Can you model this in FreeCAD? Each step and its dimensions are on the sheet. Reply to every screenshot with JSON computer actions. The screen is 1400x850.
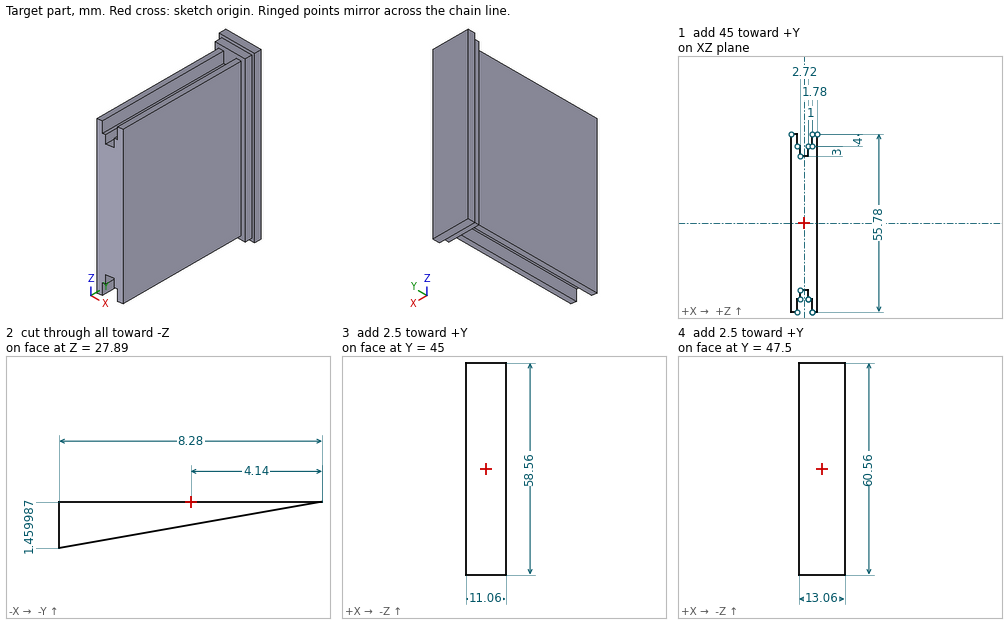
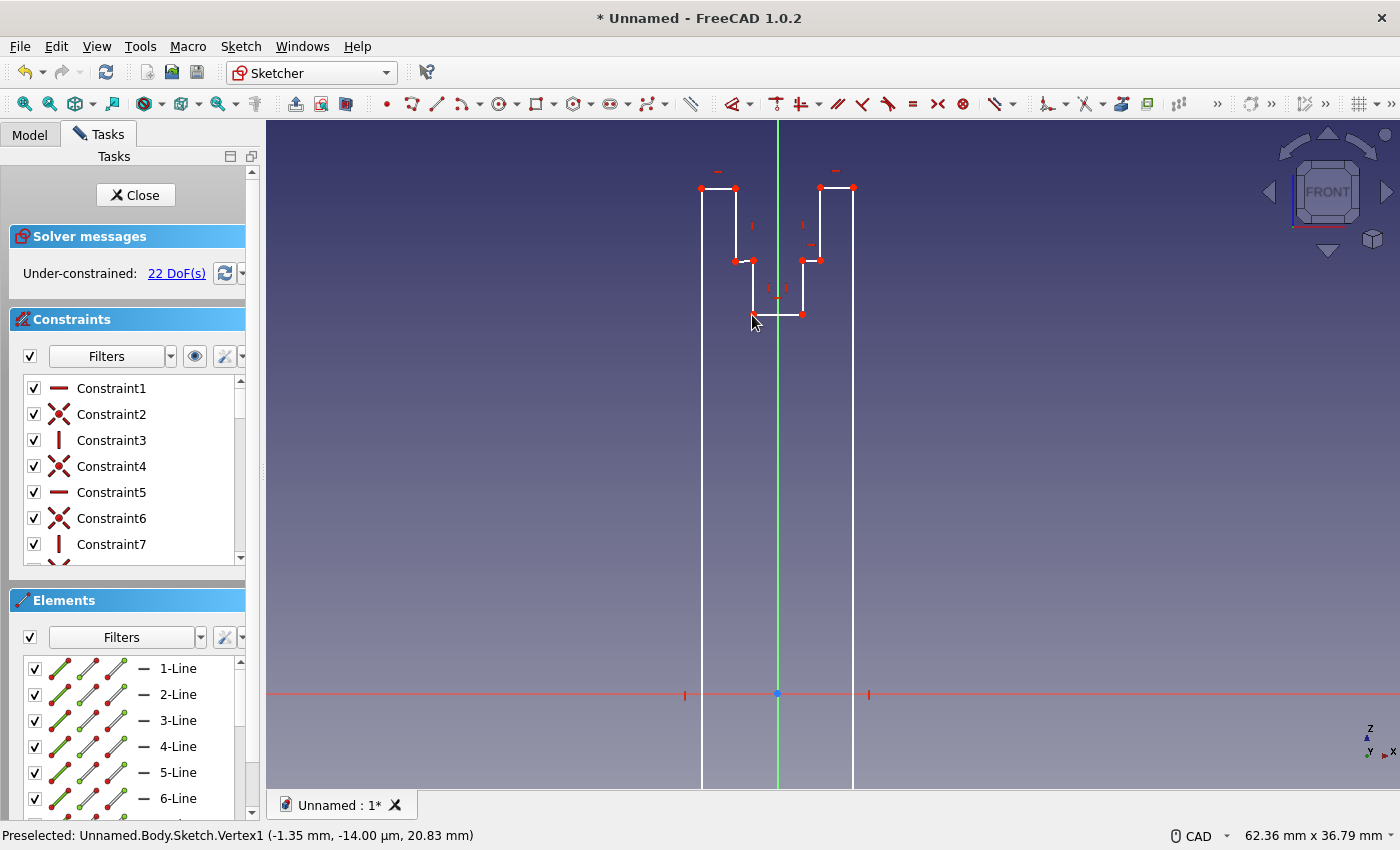
{"action": "scroll", "coordinate": [754, 259], "scroll_direction": "down", "scroll_amount": 4}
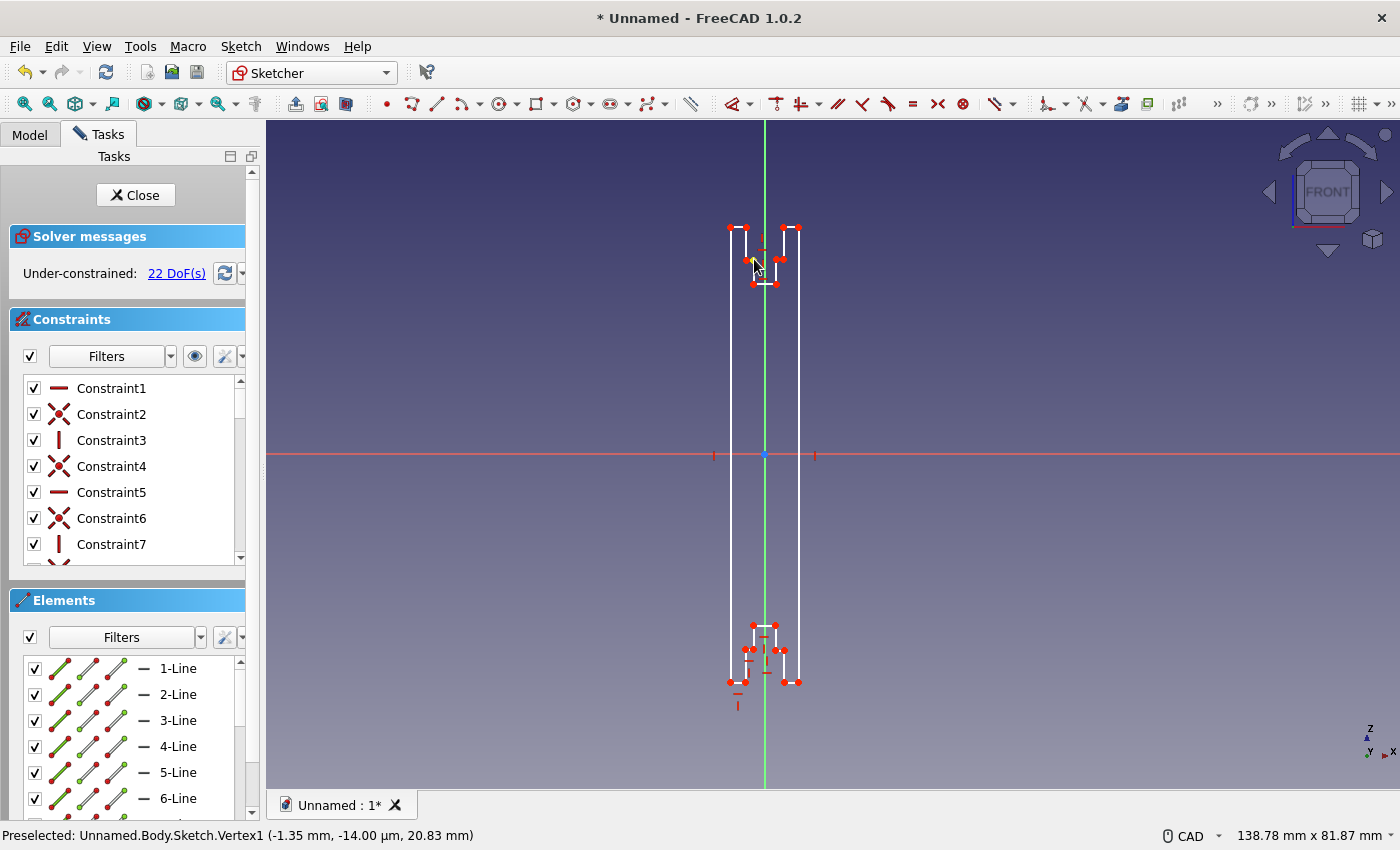
{"action": "scroll", "coordinate": [780, 651], "scroll_direction": "up", "scroll_amount": 7}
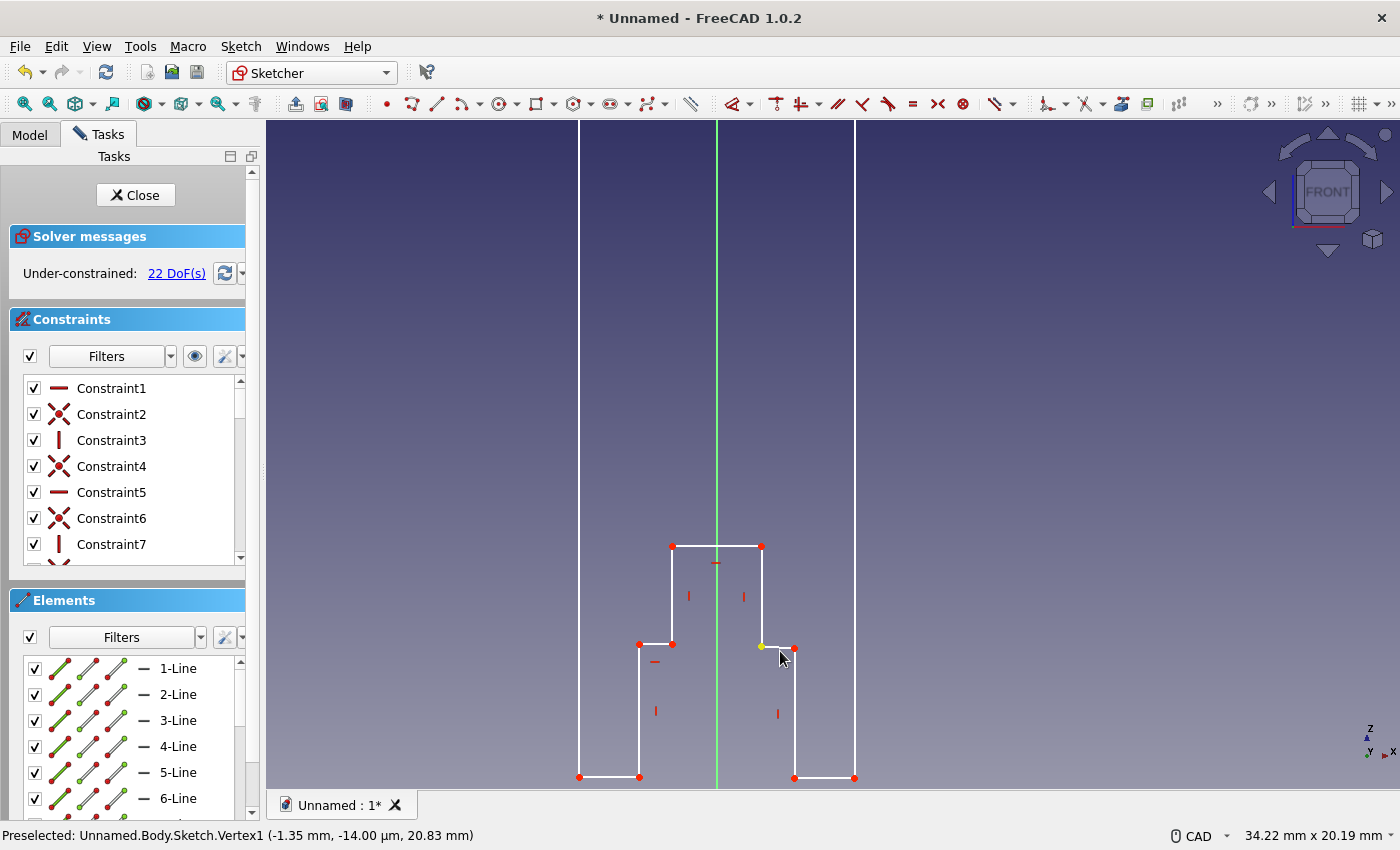
{"action": "left_click", "coordinate": [778, 647]}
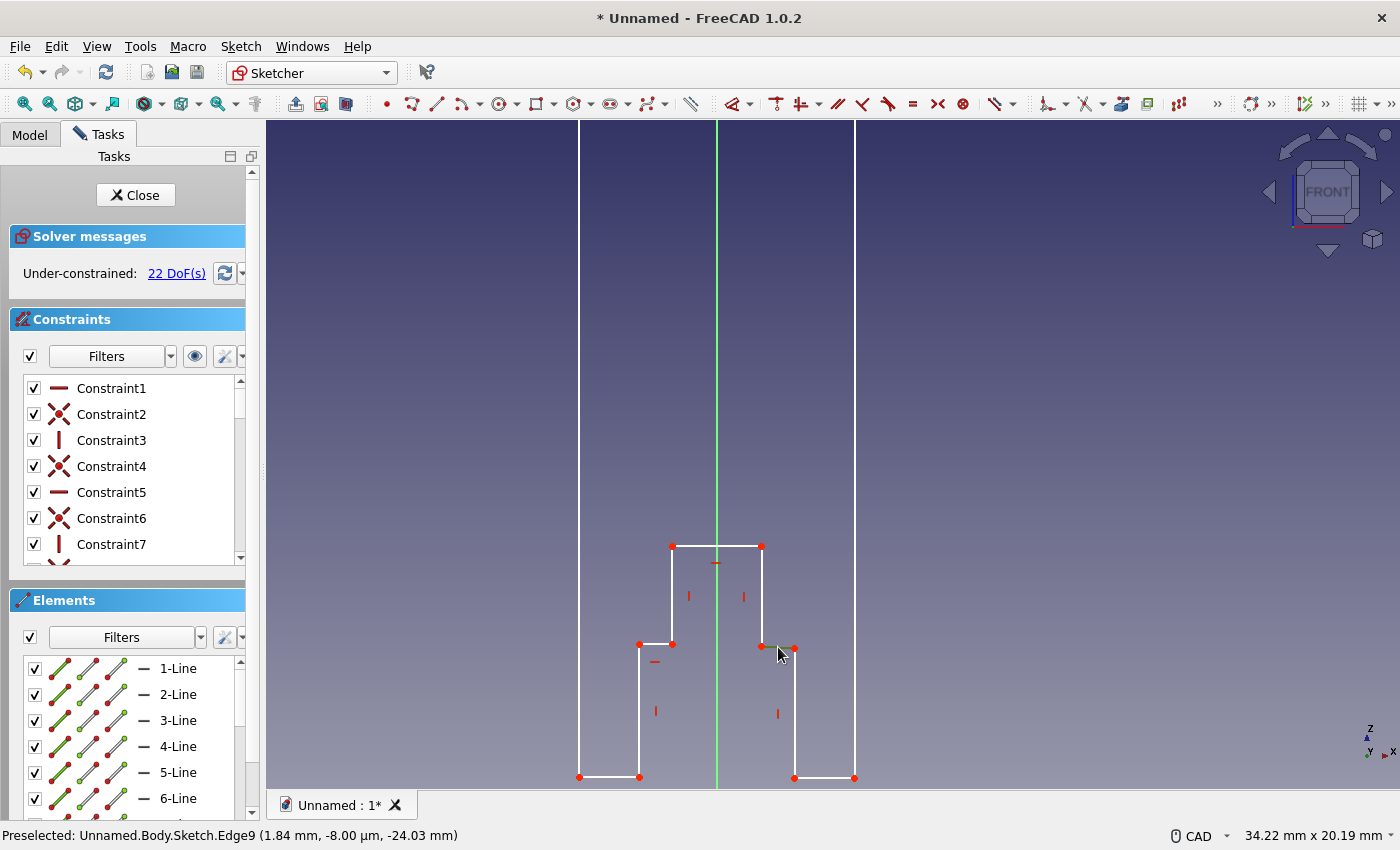
{"action": "left_click", "coordinate": [818, 104]}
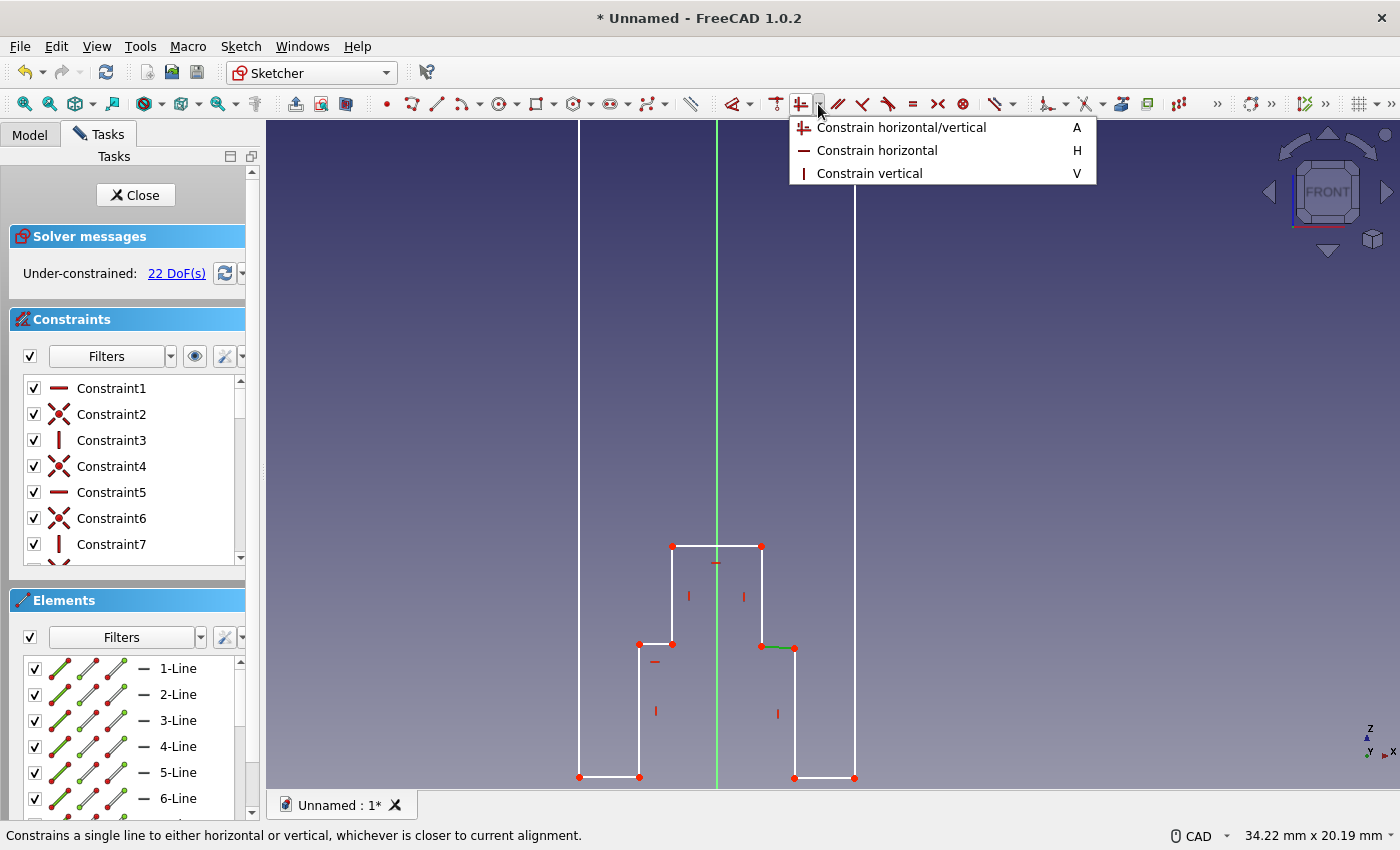
{"action": "left_click", "coordinate": [943, 150]}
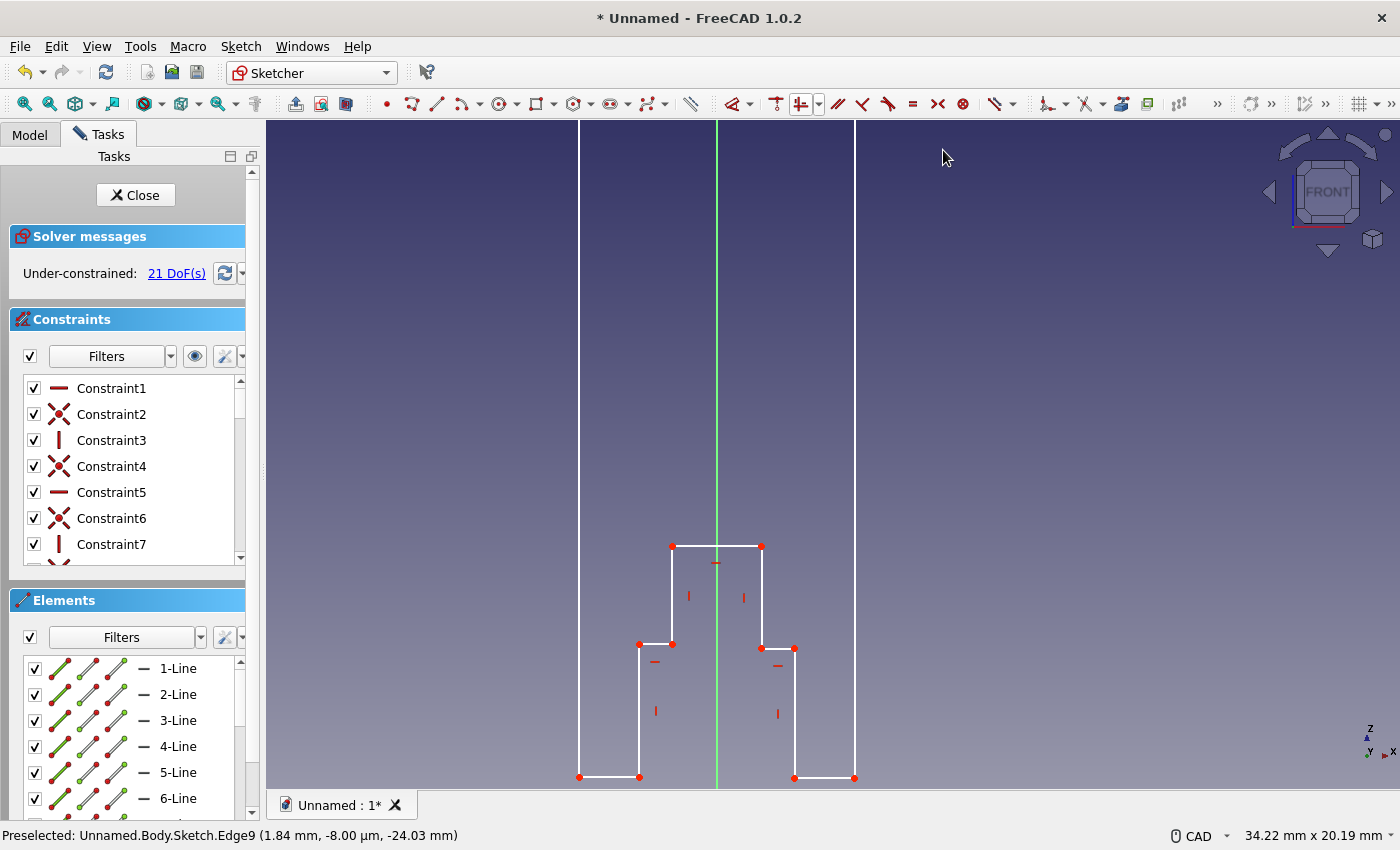
{"action": "scroll", "coordinate": [780, 652], "scroll_direction": "down", "scroll_amount": 7}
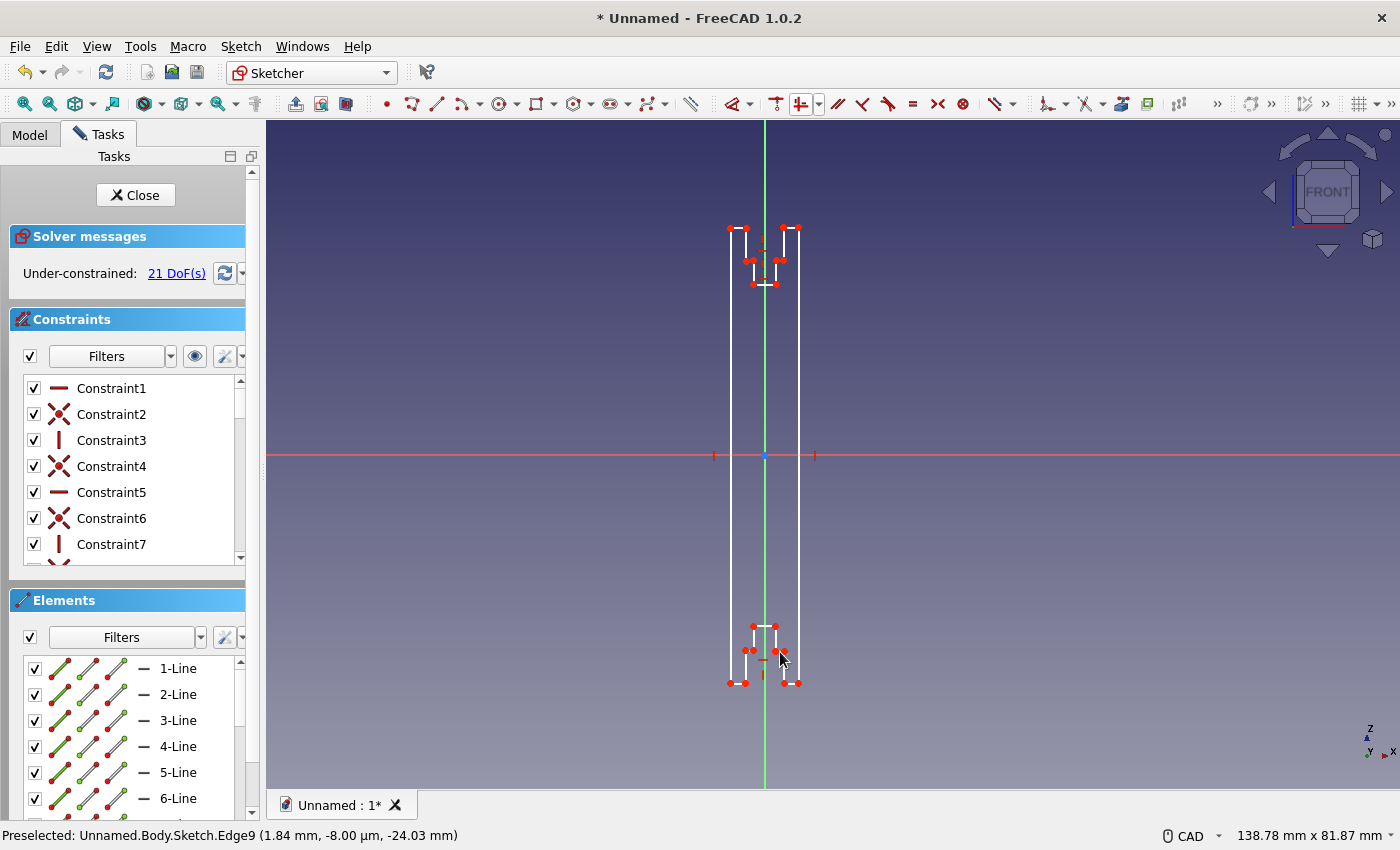
{"action": "scroll", "coordinate": [748, 261], "scroll_direction": "up", "scroll_amount": 9}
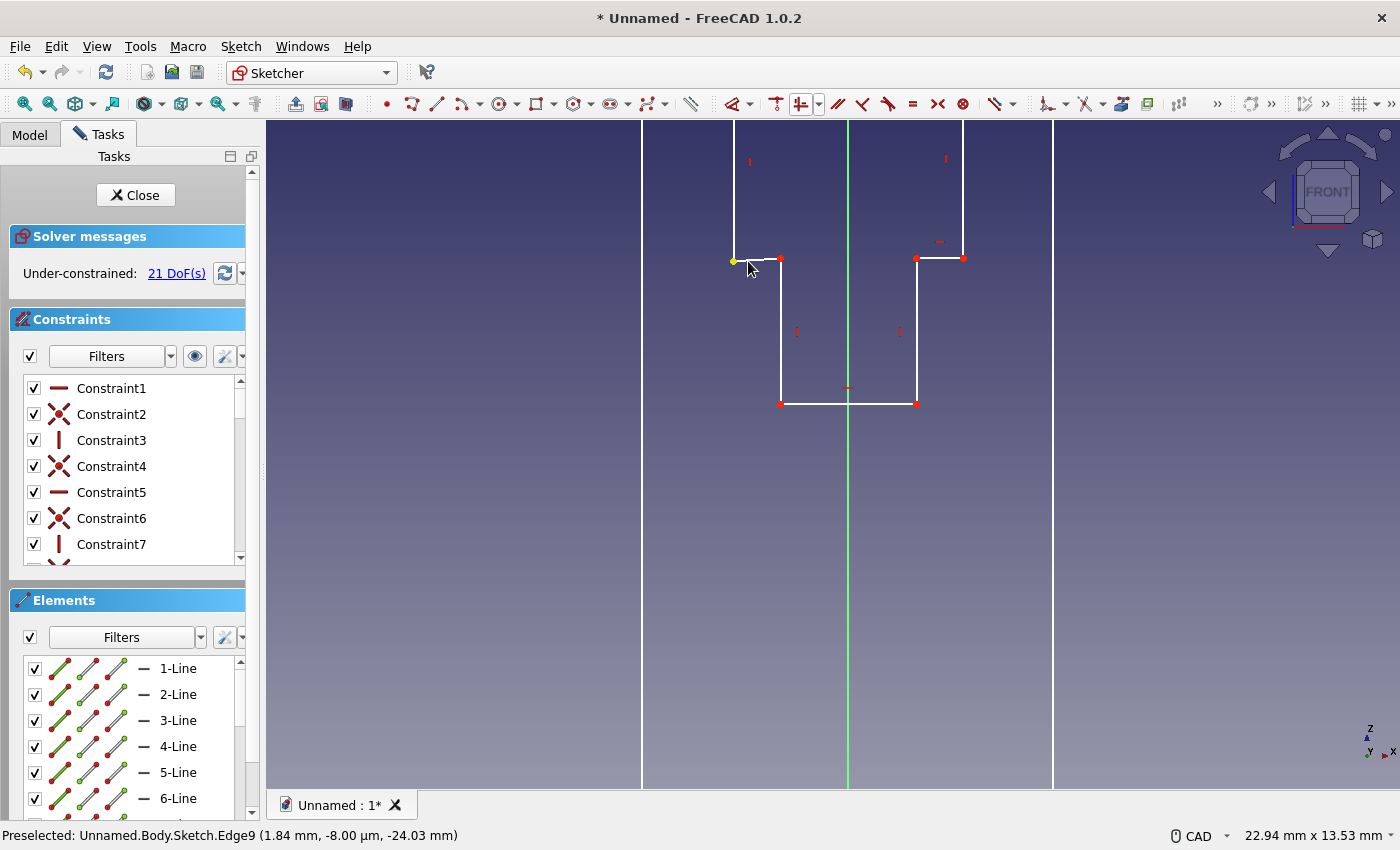
{"action": "left_click", "coordinate": [748, 260]}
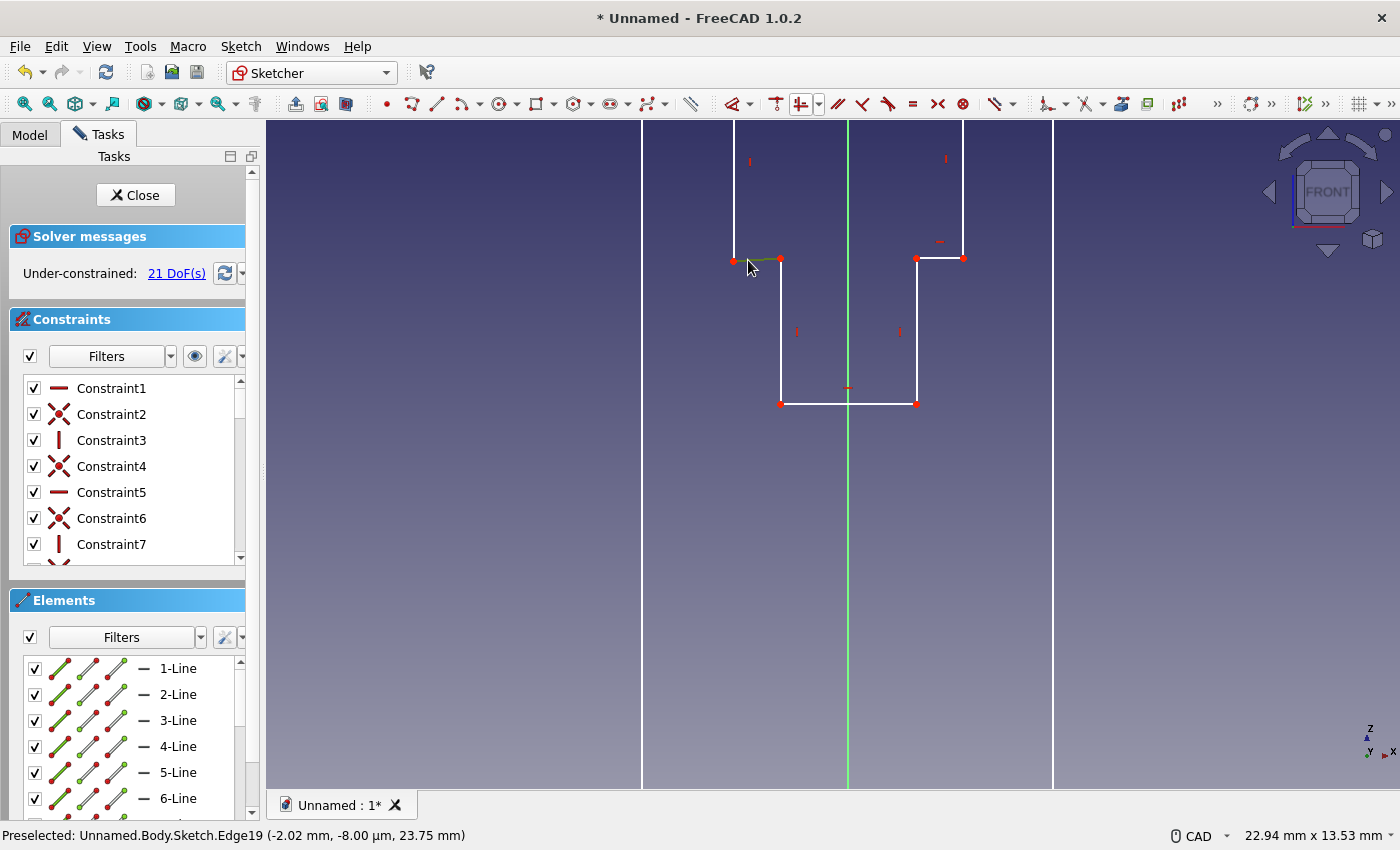
{"action": "key", "text": "h"}